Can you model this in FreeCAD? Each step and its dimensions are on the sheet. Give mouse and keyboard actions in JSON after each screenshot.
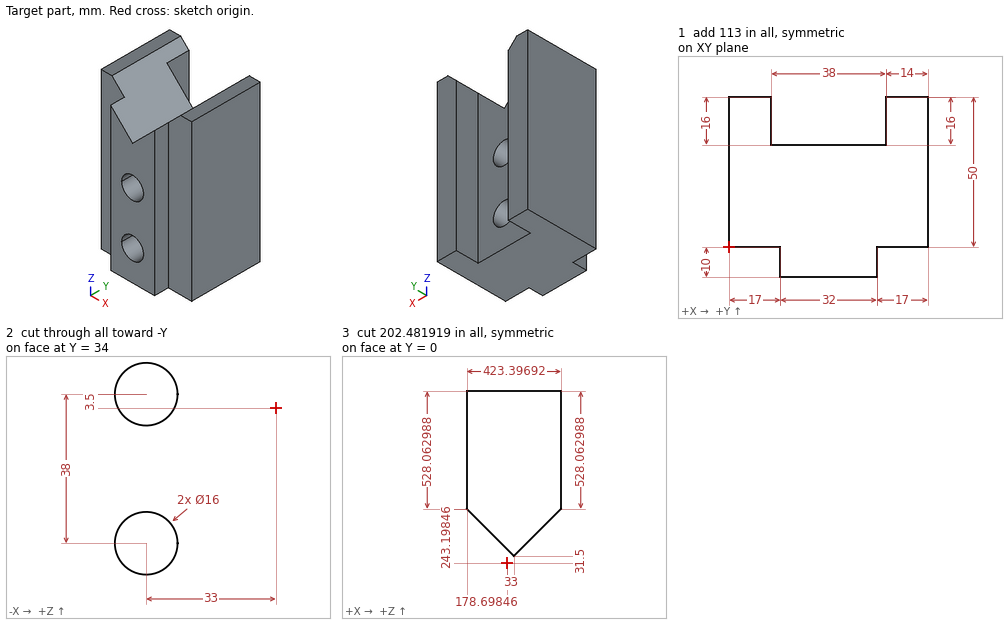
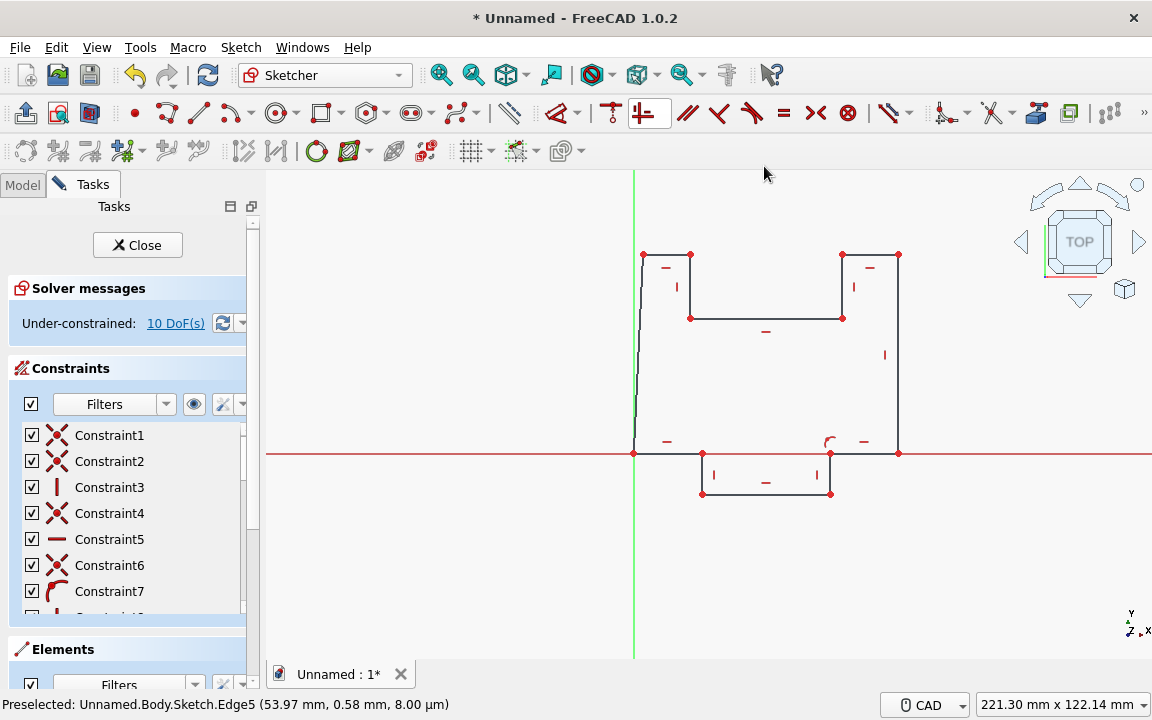
{"action": "left_click", "coordinate": [637, 394]}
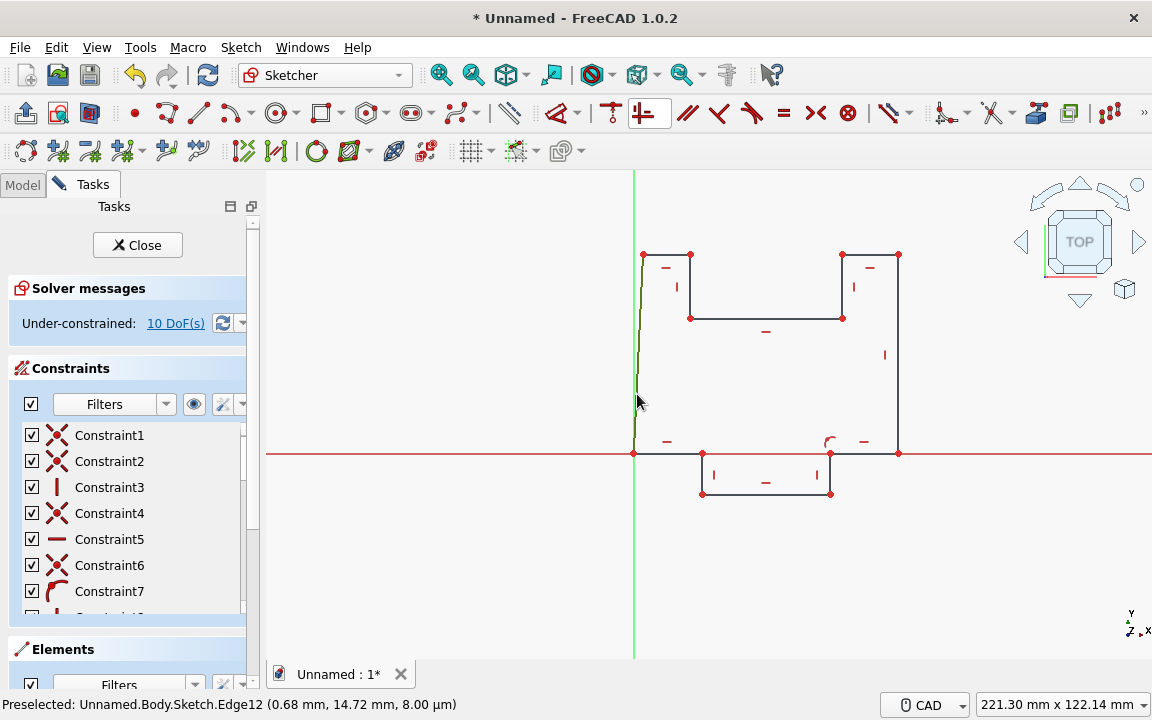
{"action": "left_click", "coordinate": [666, 114]}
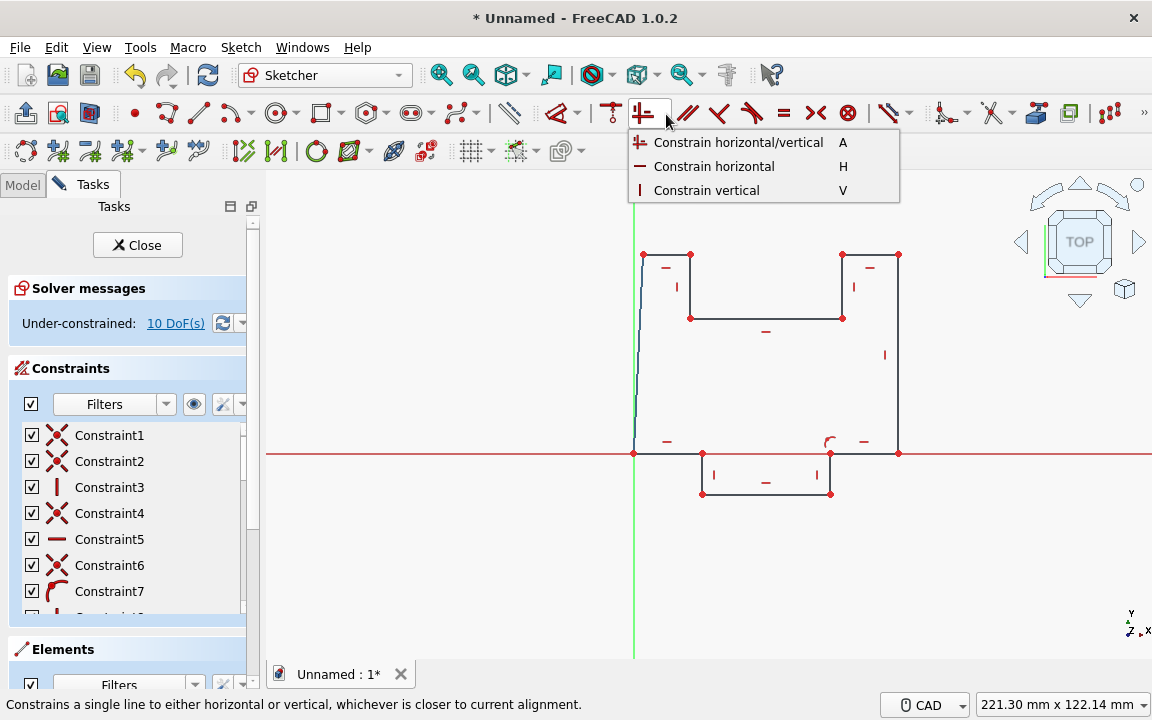
{"action": "left_click", "coordinate": [764, 190]}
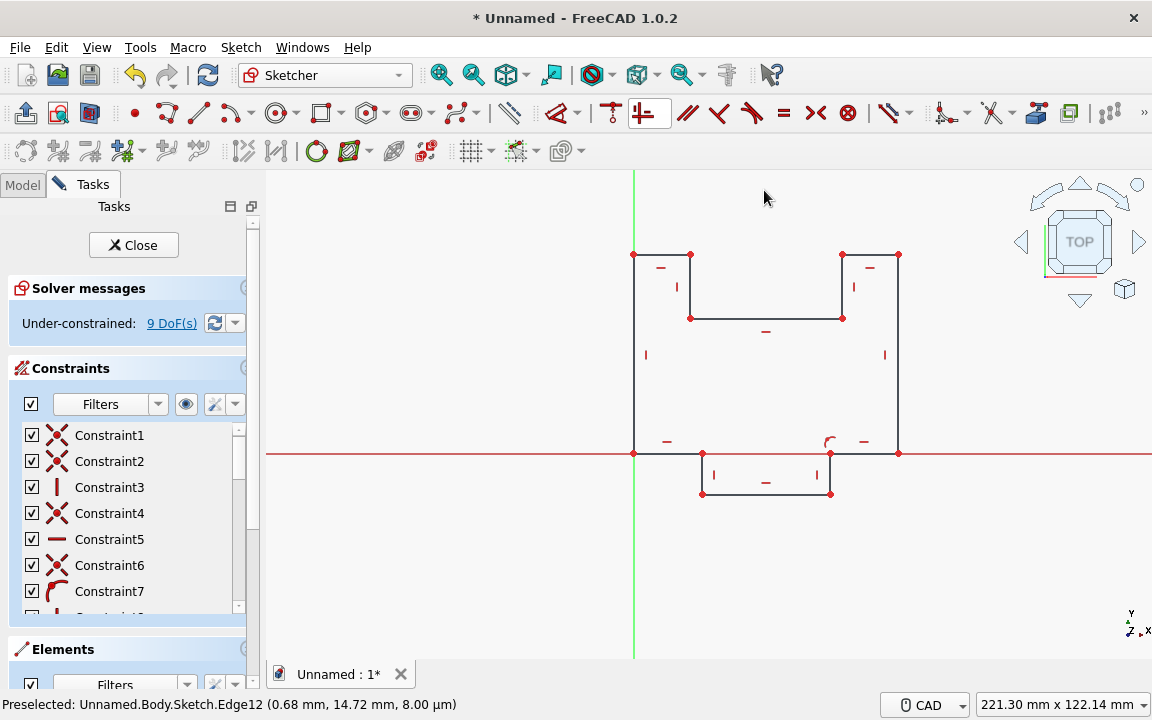
{"action": "left_click", "coordinate": [556, 114]}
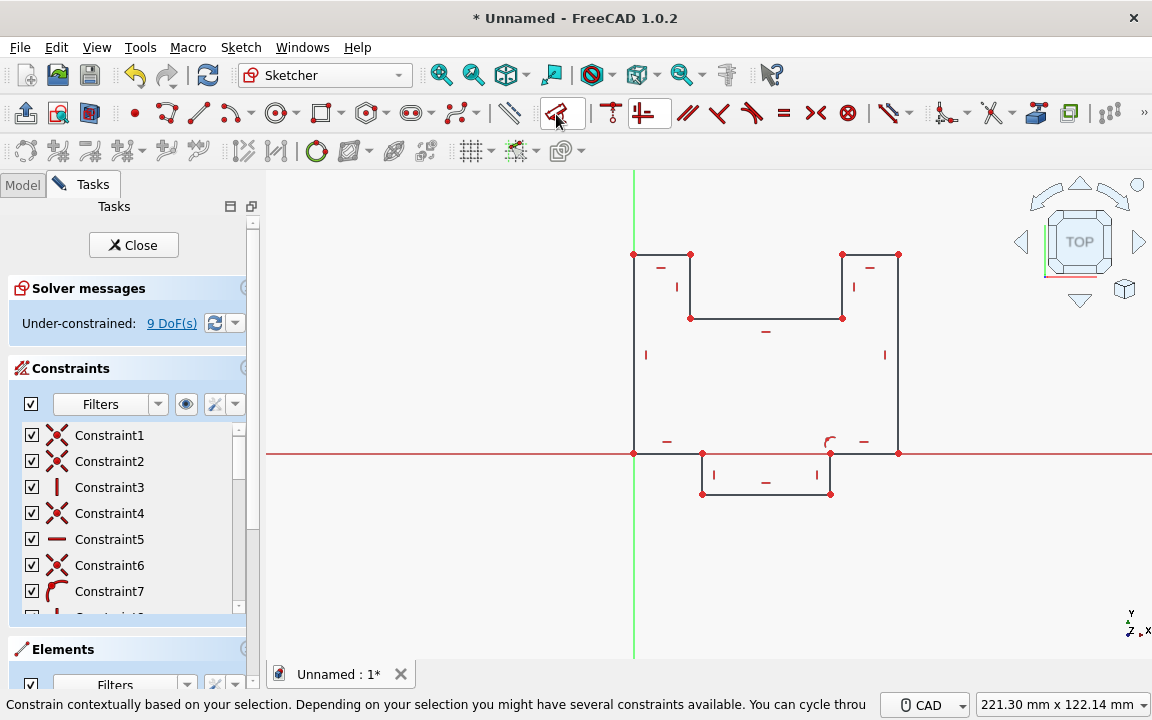
{"action": "left_click", "coordinate": [654, 454]}
{"action": "left_click", "coordinate": [668, 488]}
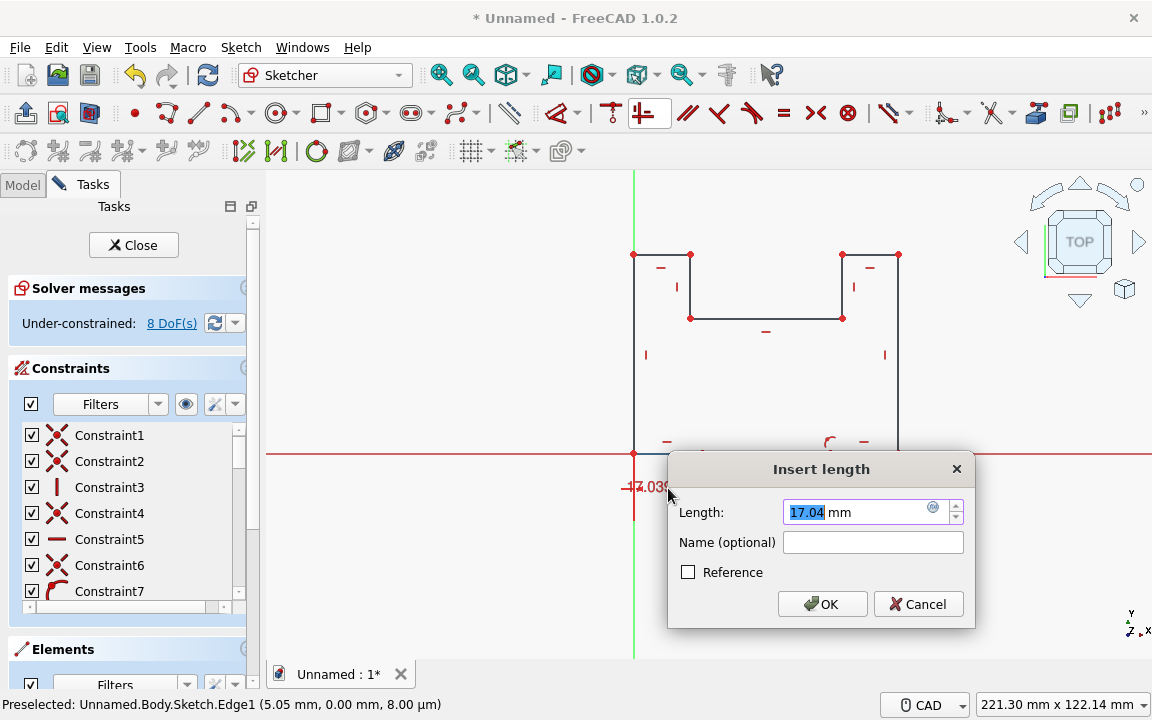
{"action": "type", "text": "17"}
{"action": "key", "text": "Return"}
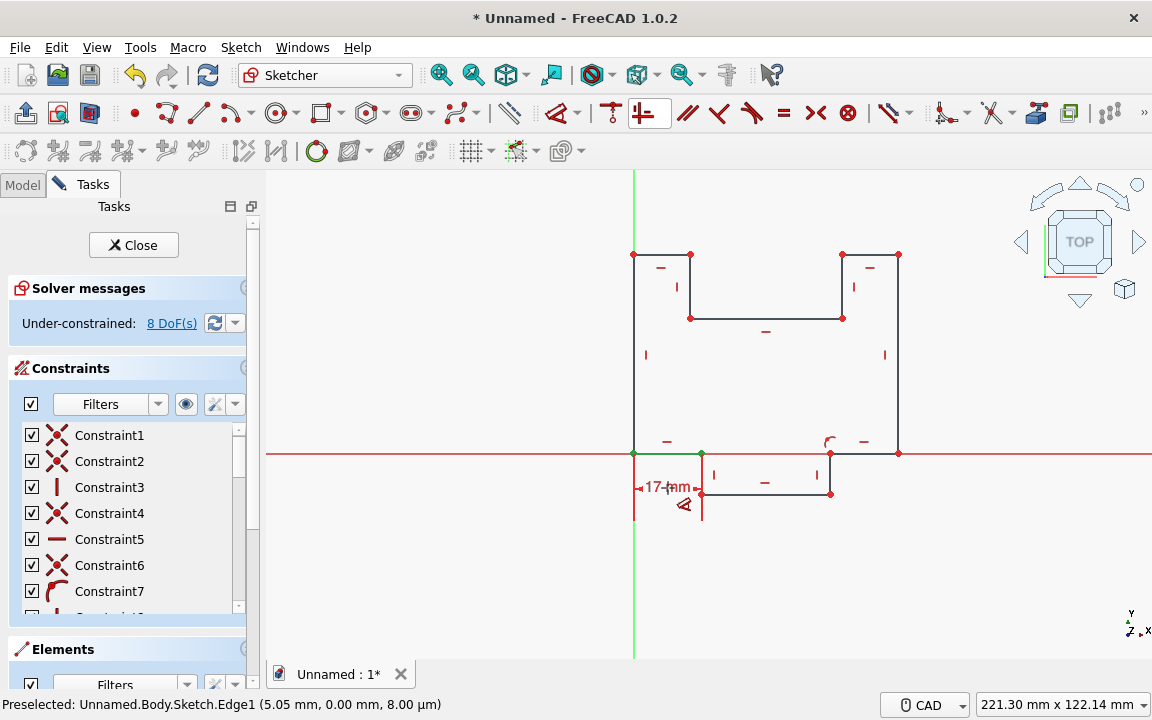
{"action": "left_click", "coordinate": [702, 466]}
{"action": "left_click", "coordinate": [760, 474]}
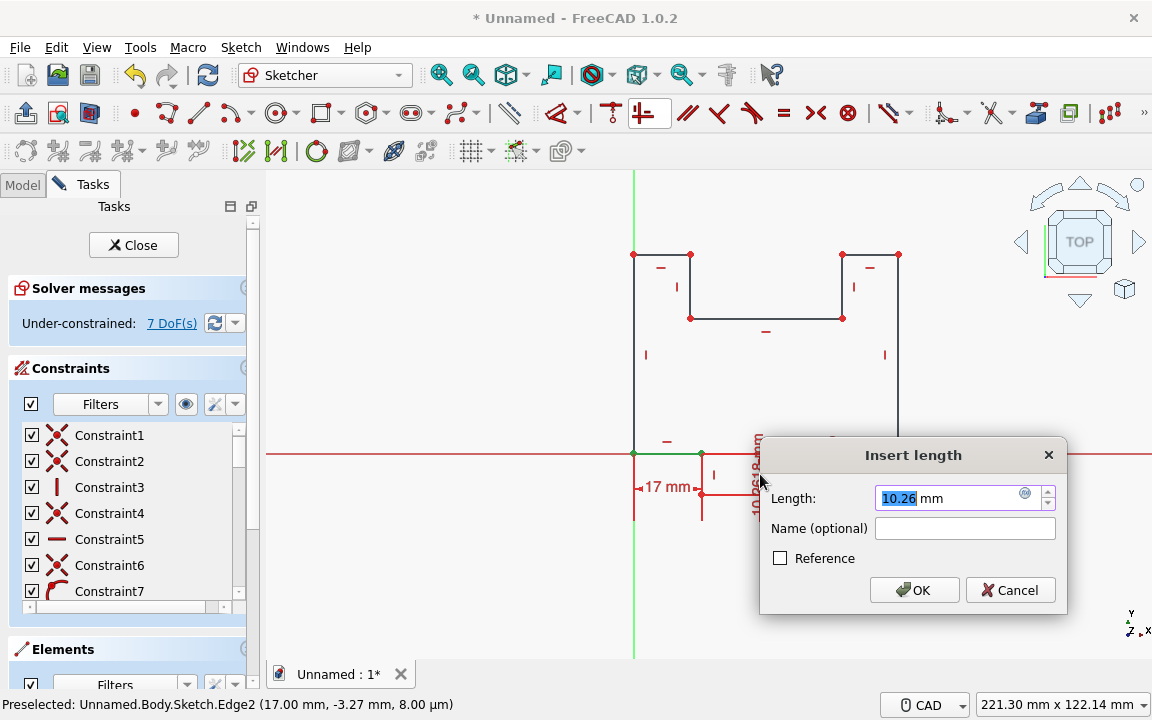
{"action": "type", "text": "10"}
{"action": "key", "text": "Return"}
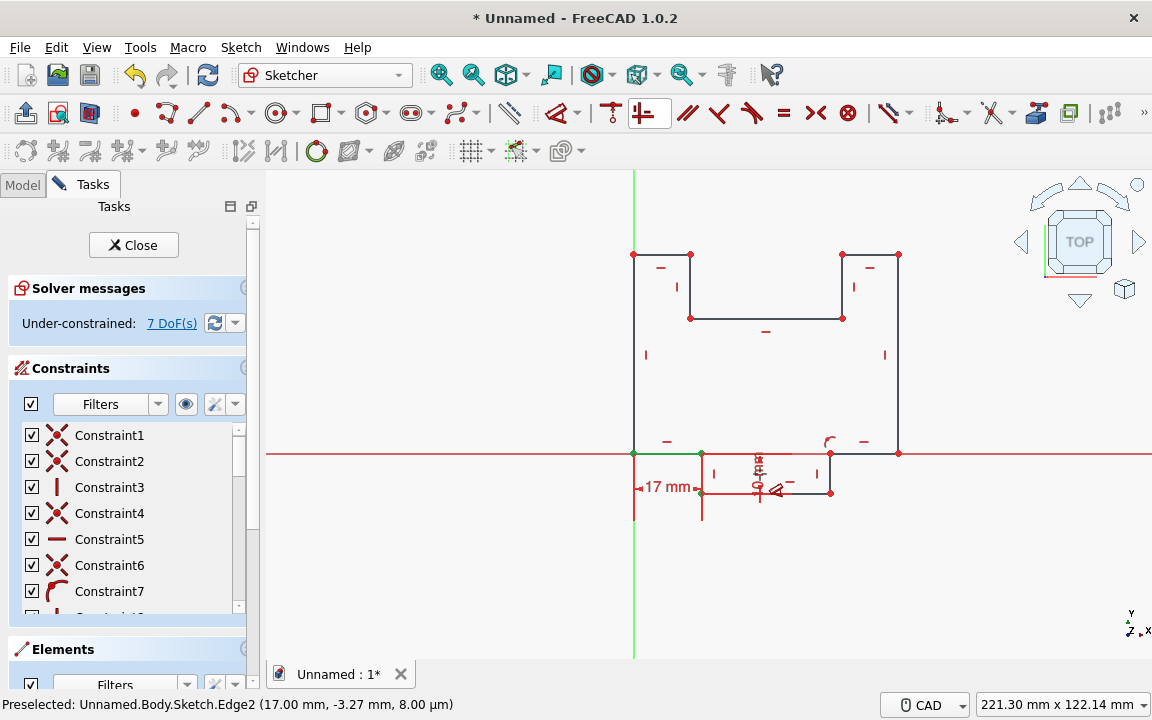
{"action": "left_click", "coordinate": [740, 494]}
{"action": "left_click", "coordinate": [766, 528]}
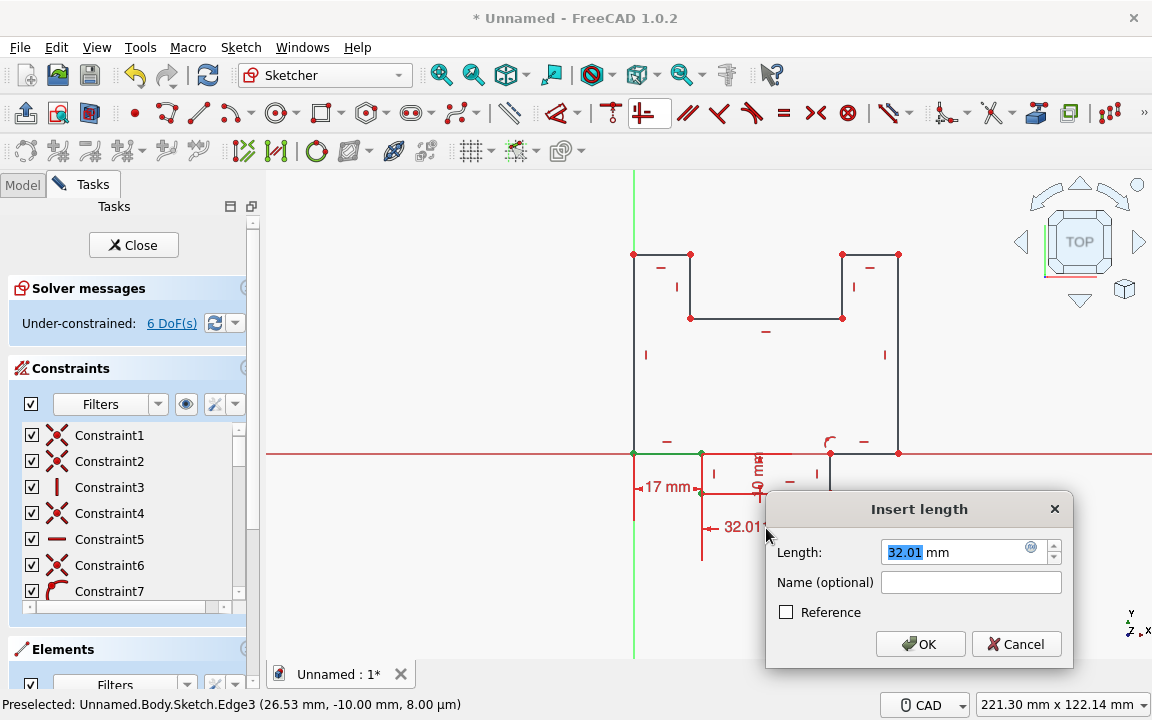
{"action": "type", "text": "32"}
{"action": "key", "text": "Return"}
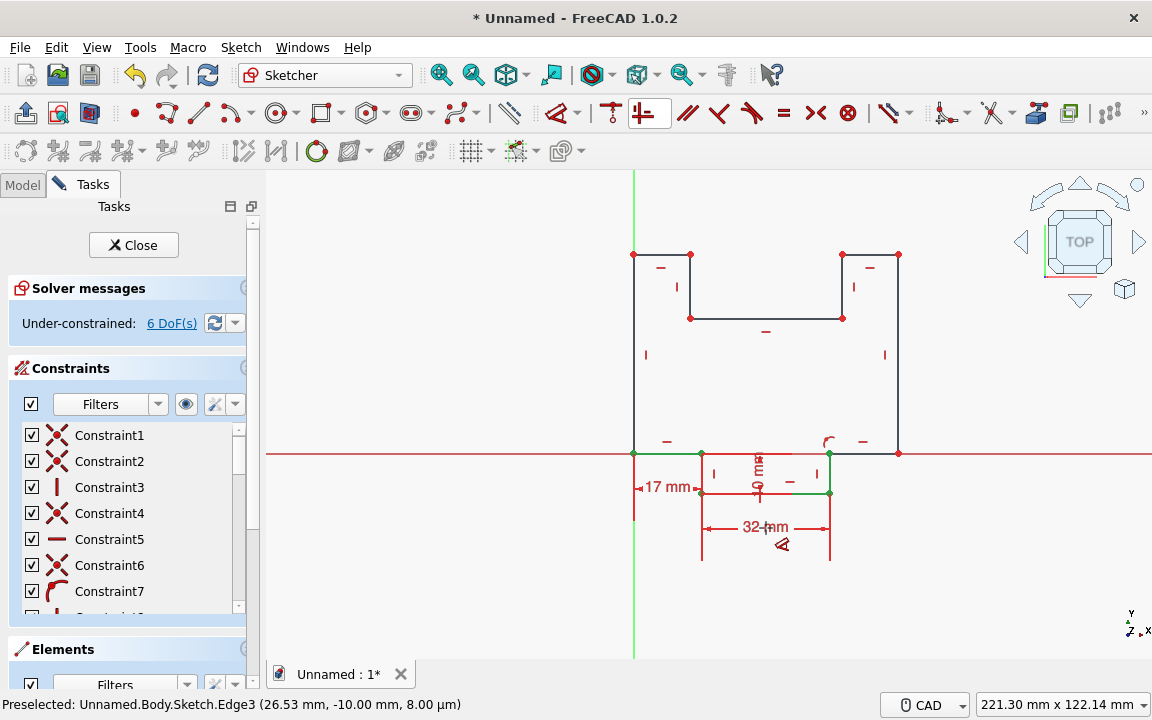
{"action": "left_click", "coordinate": [850, 454]}
{"action": "left_click", "coordinate": [864, 488]}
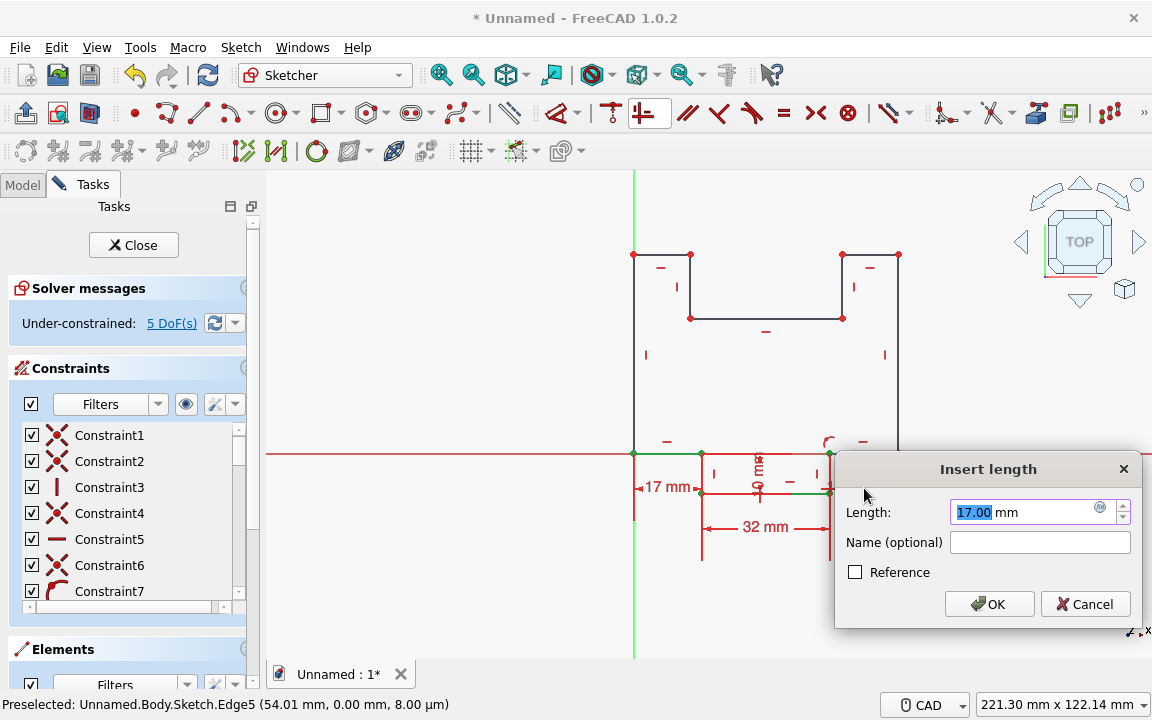
{"action": "type", "text": "17"}
{"action": "key", "text": "Return"}